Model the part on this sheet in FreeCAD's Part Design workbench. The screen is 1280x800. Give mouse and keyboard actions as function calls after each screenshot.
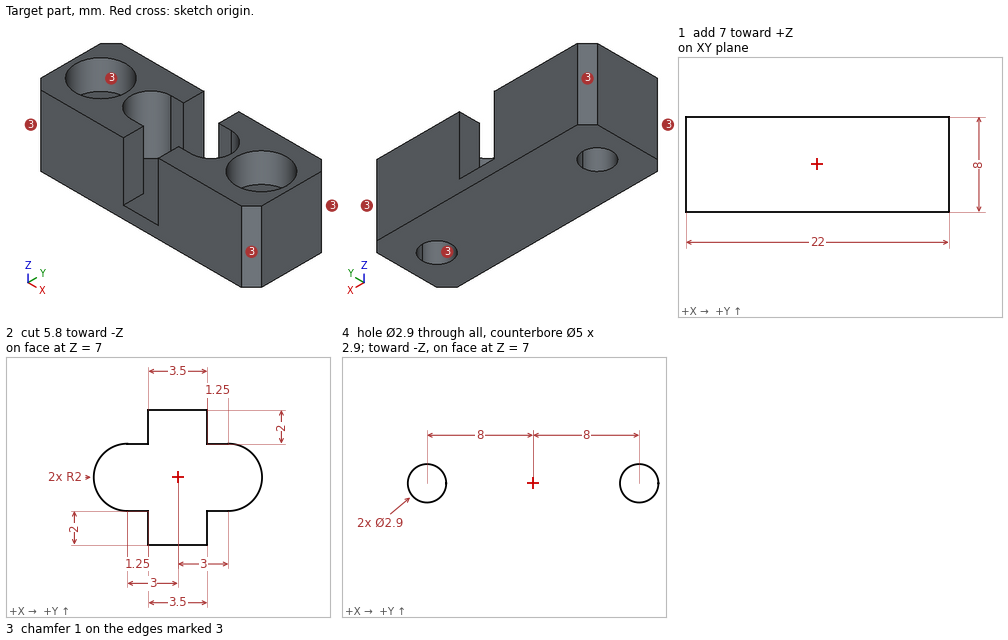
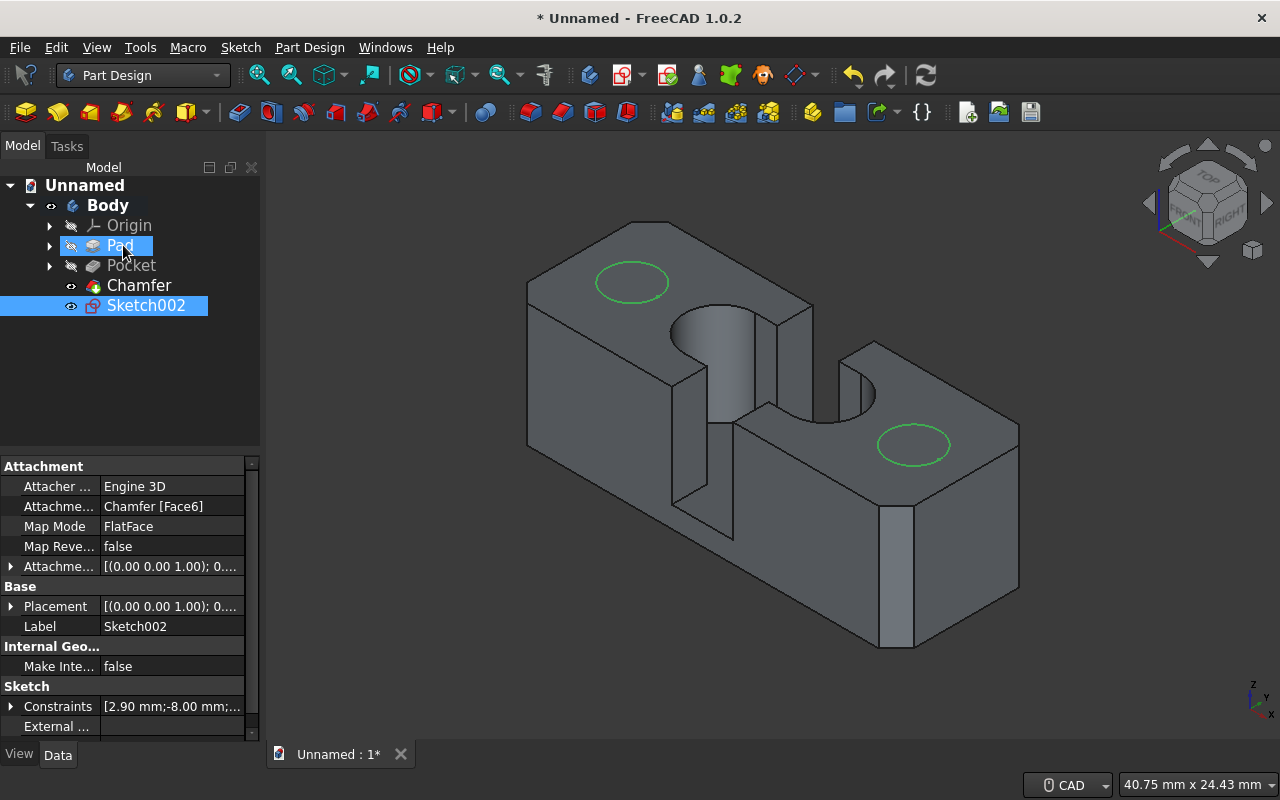
click(272, 112)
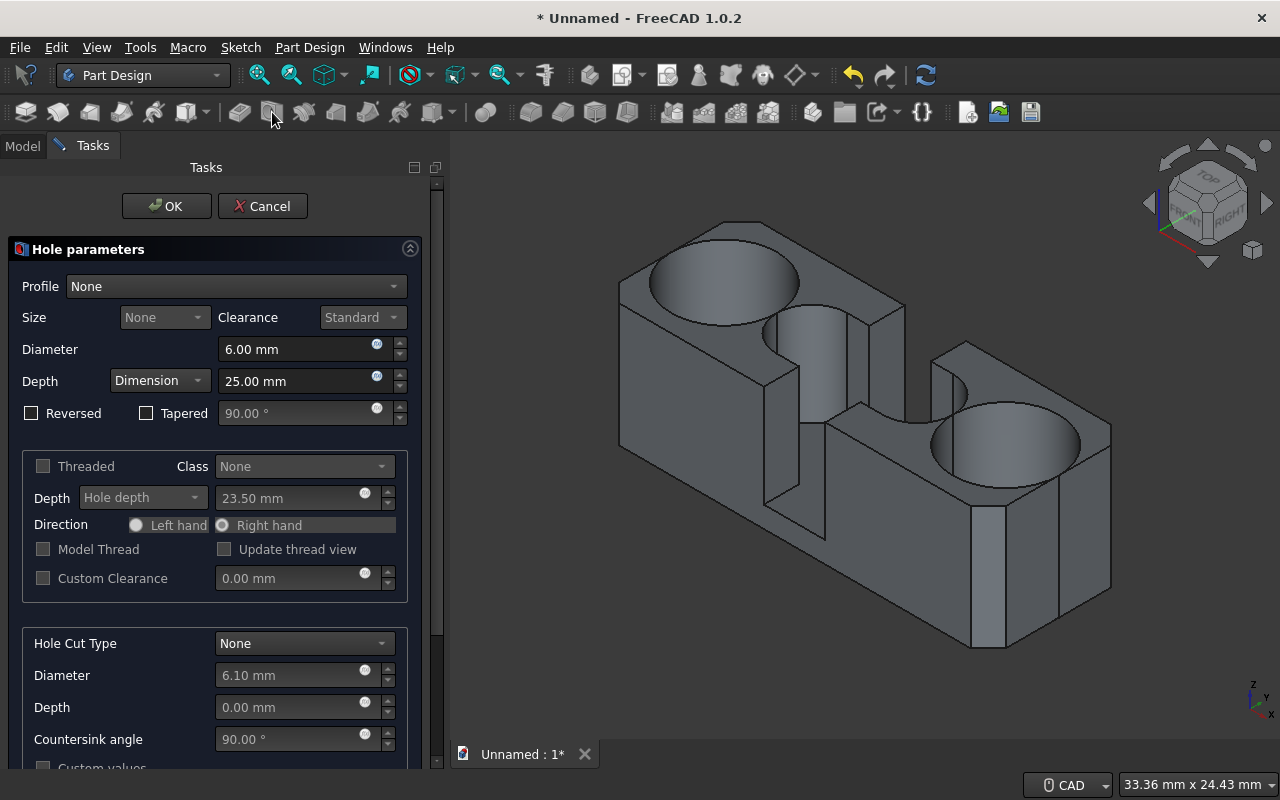
triple_click(305, 349)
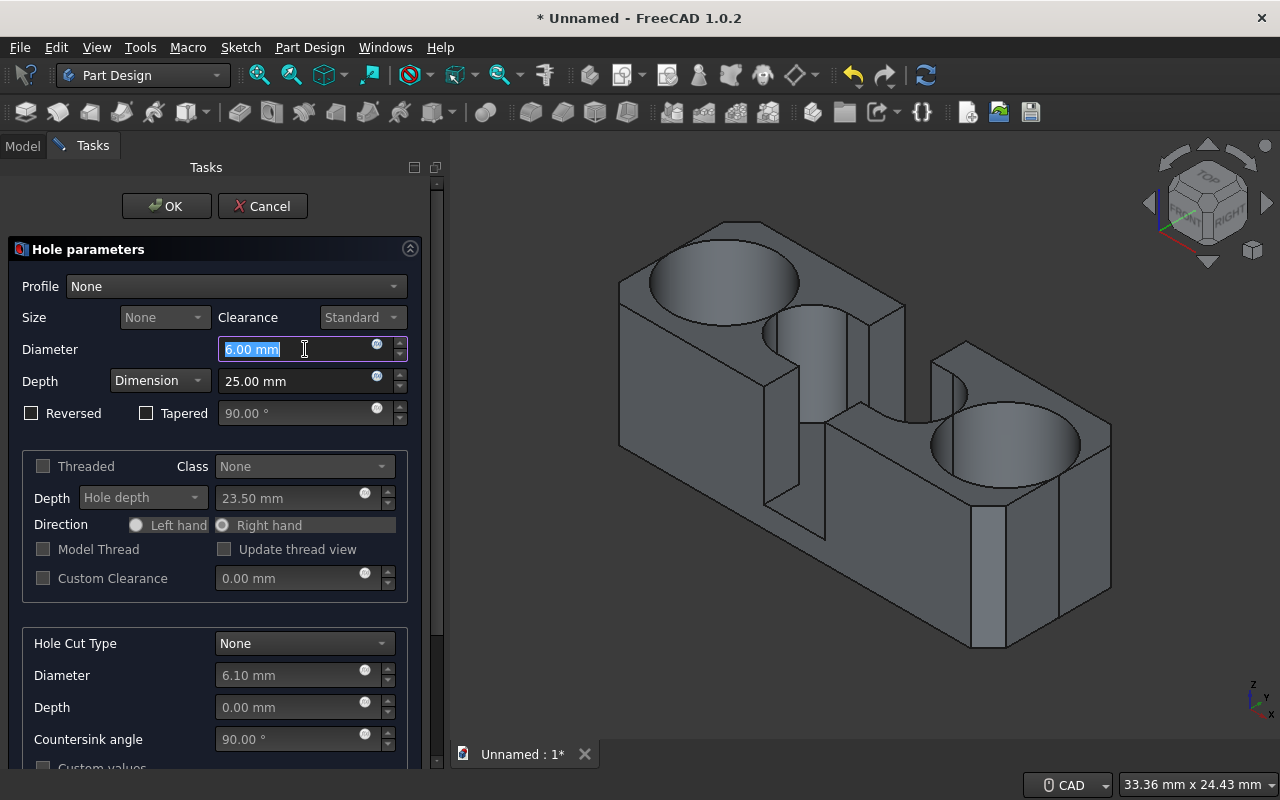
text(2.9)
key(Tab)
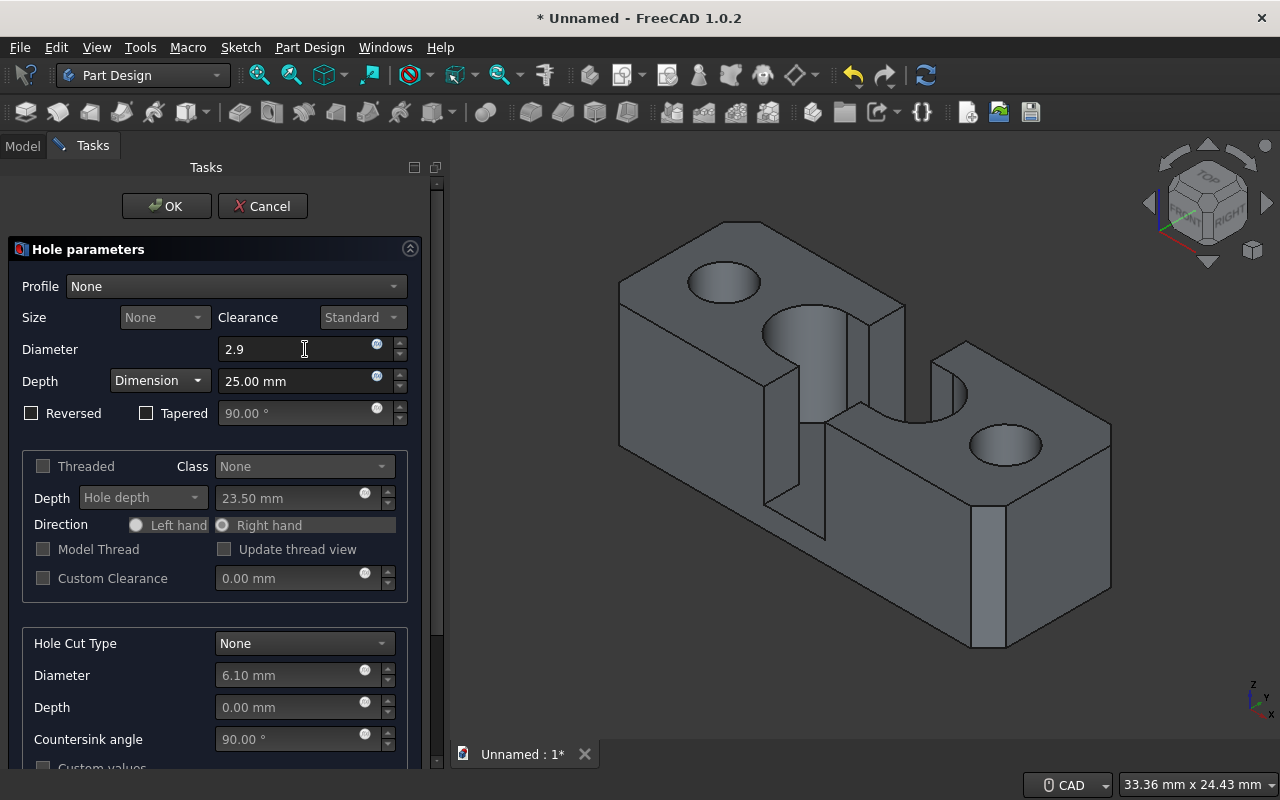
click(161, 380)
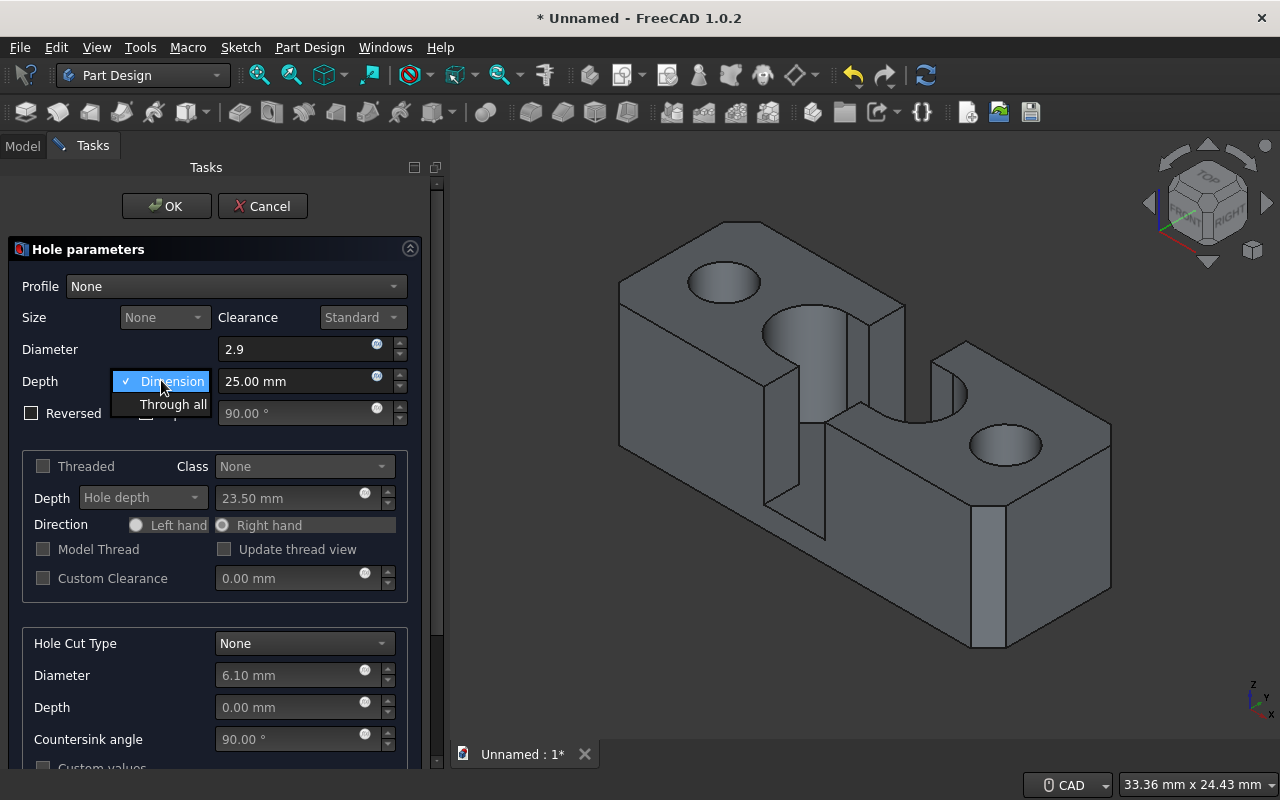
click(160, 404)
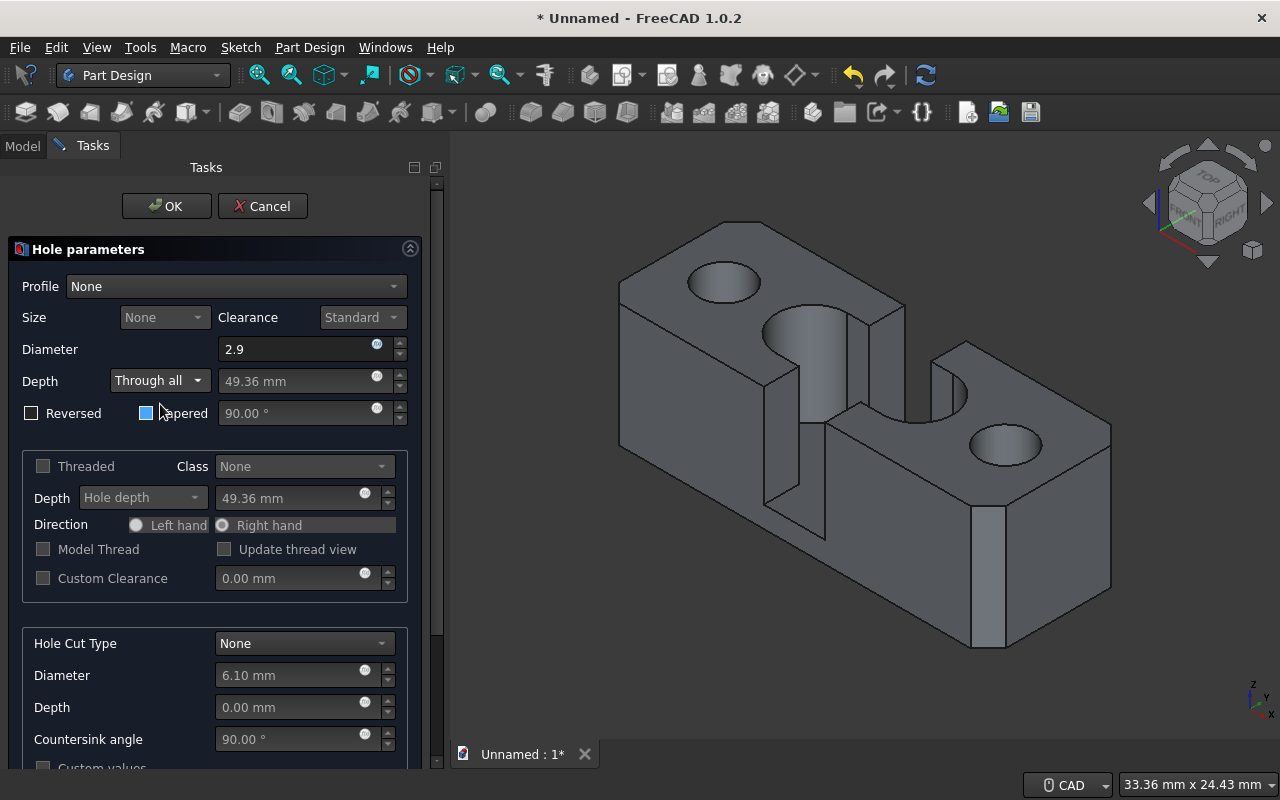
click(306, 644)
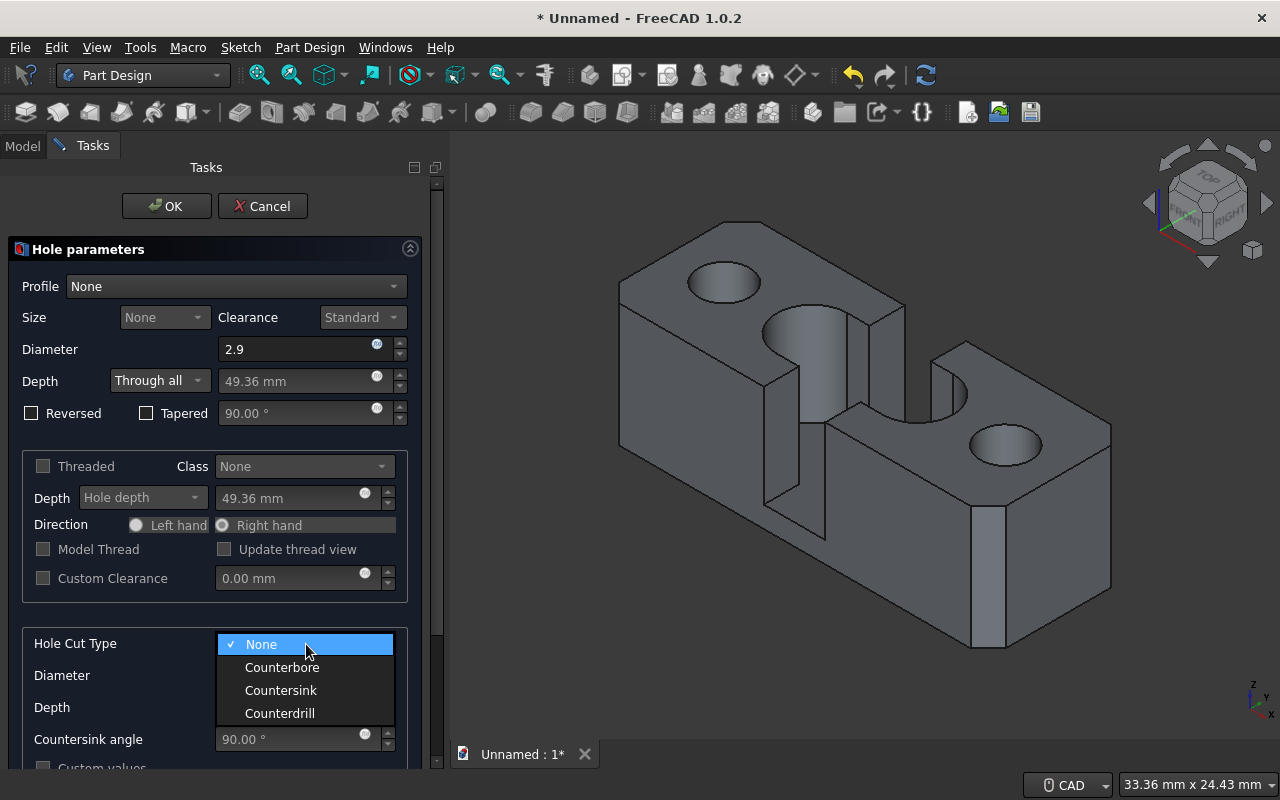
click(304, 668)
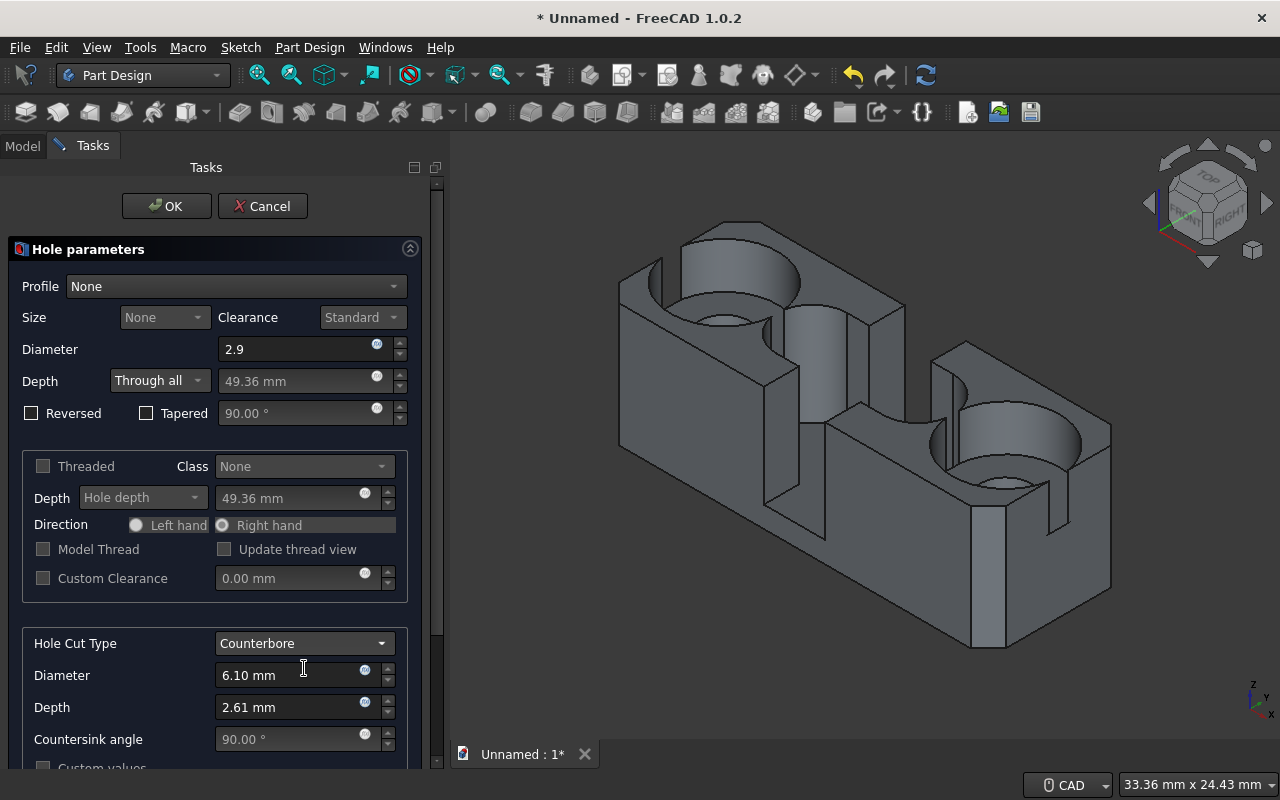
triple_click(298, 675)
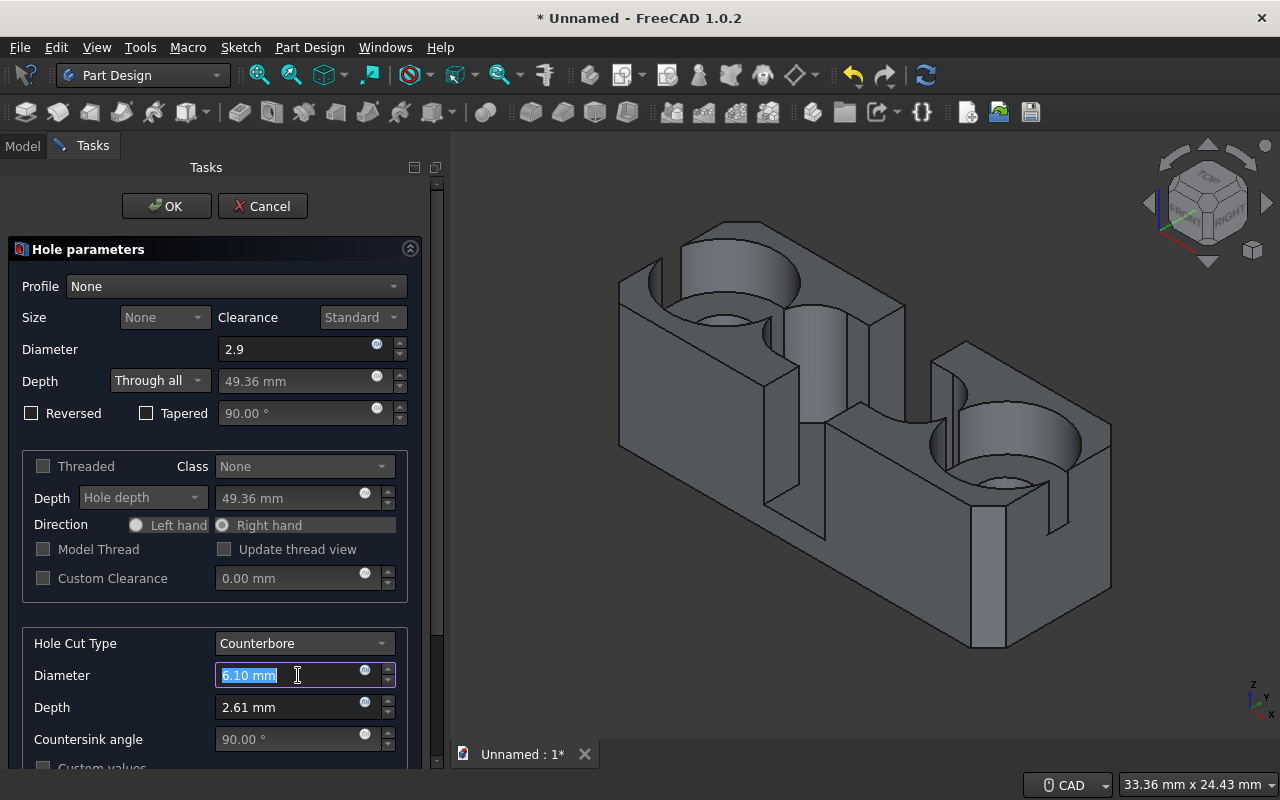
text(5)
key(Tab)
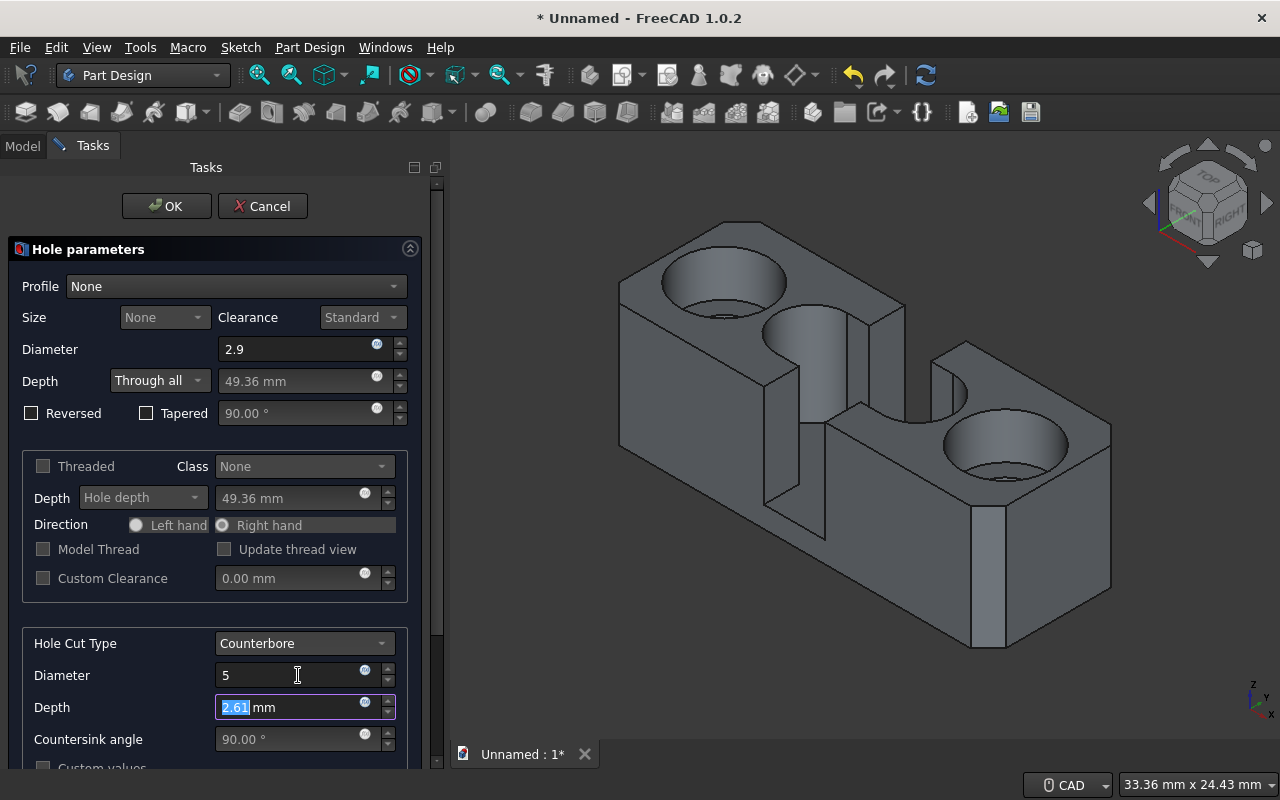
text(2.9)
key(Tab)